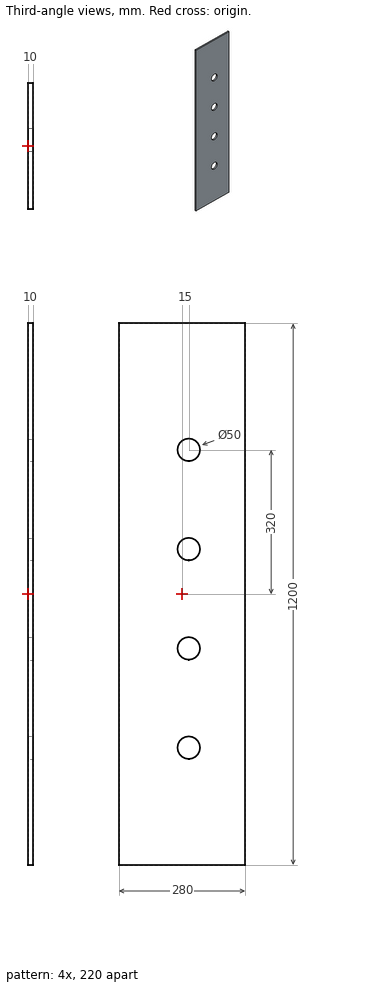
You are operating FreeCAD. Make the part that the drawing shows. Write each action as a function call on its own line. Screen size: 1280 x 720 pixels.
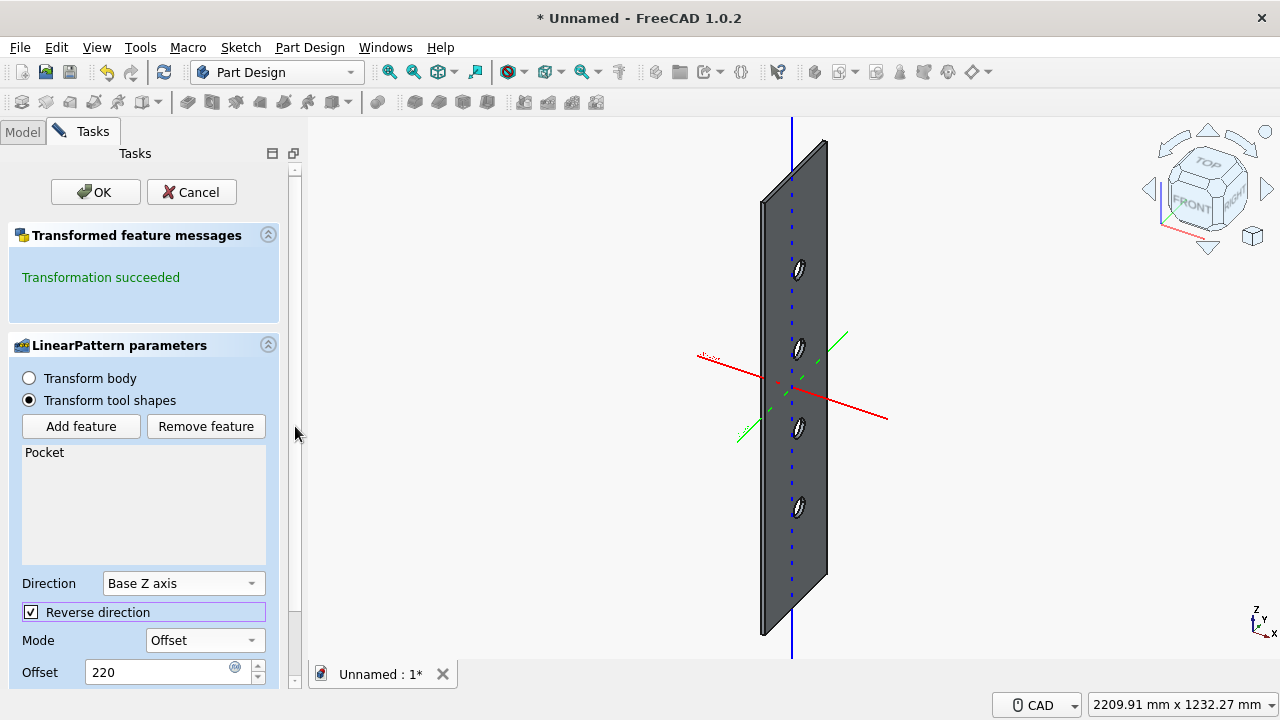
click(96, 192)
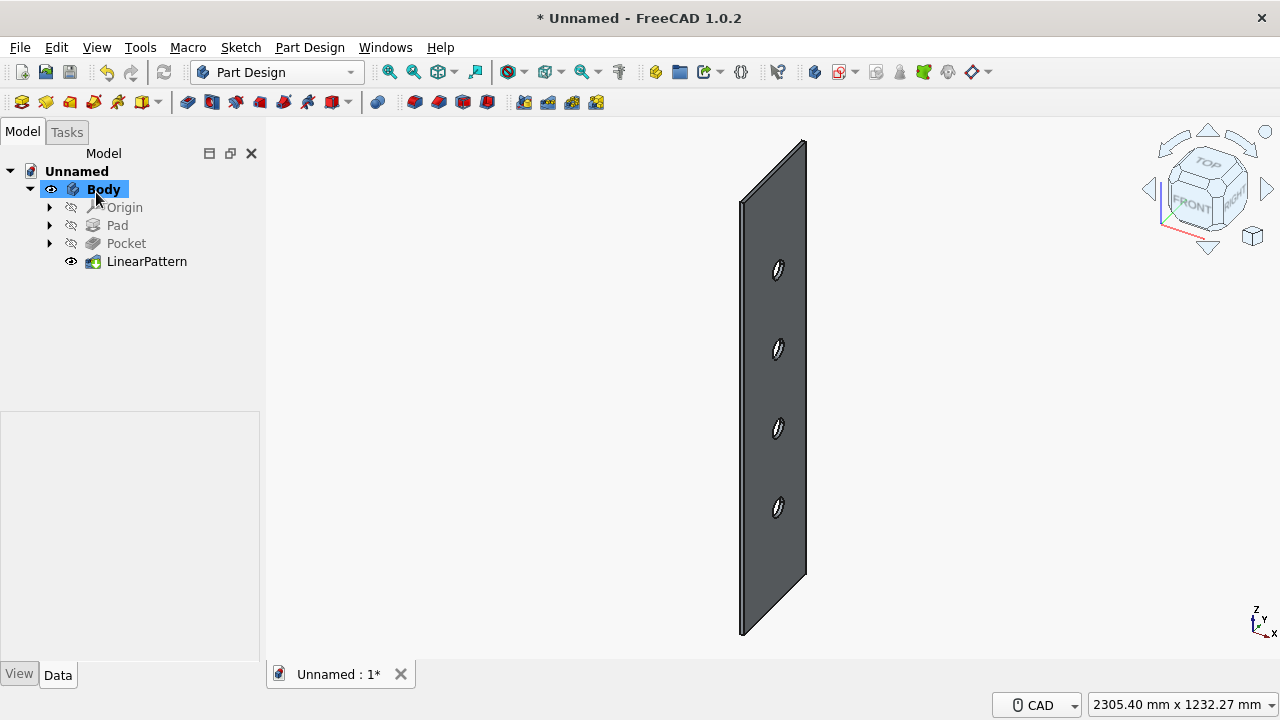
key(0)